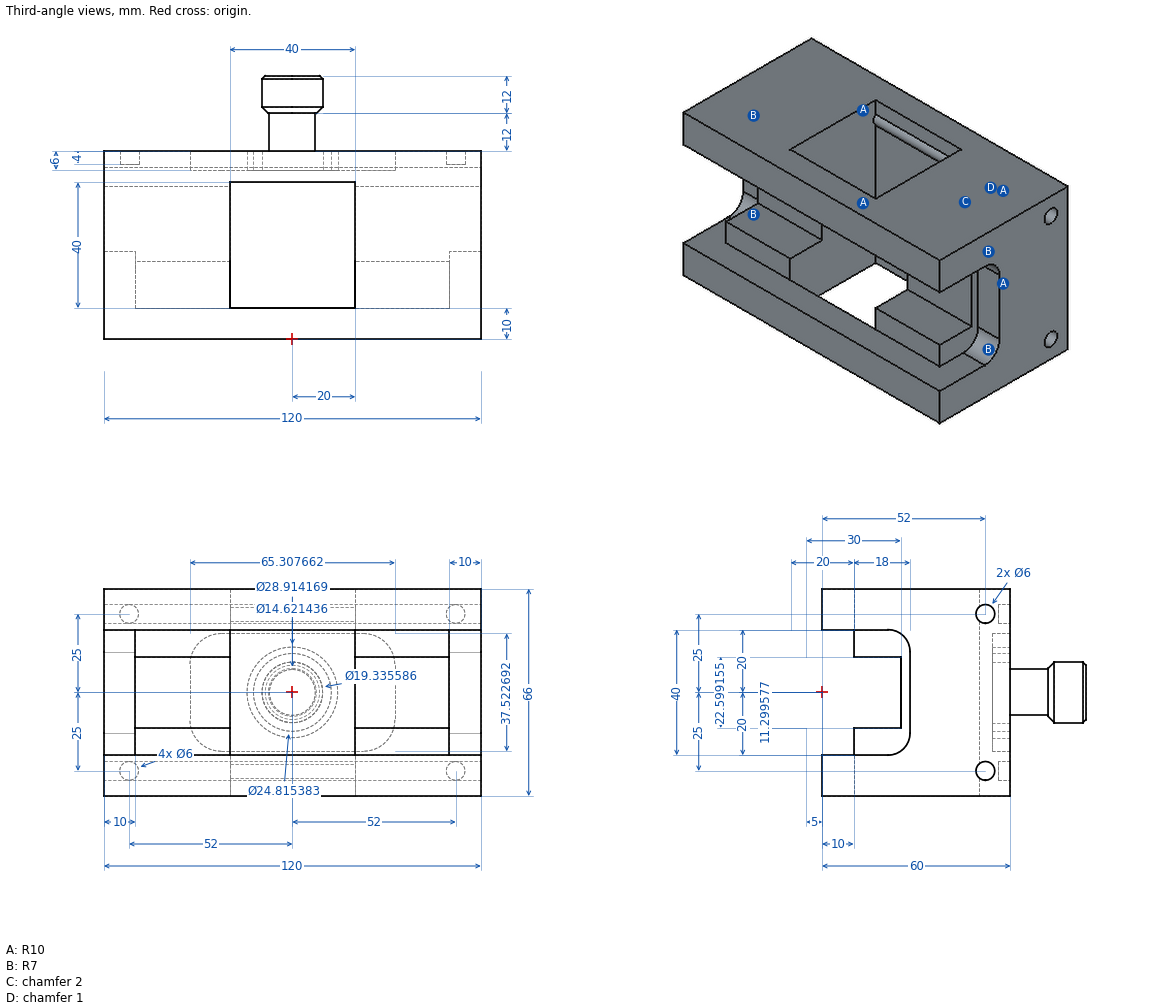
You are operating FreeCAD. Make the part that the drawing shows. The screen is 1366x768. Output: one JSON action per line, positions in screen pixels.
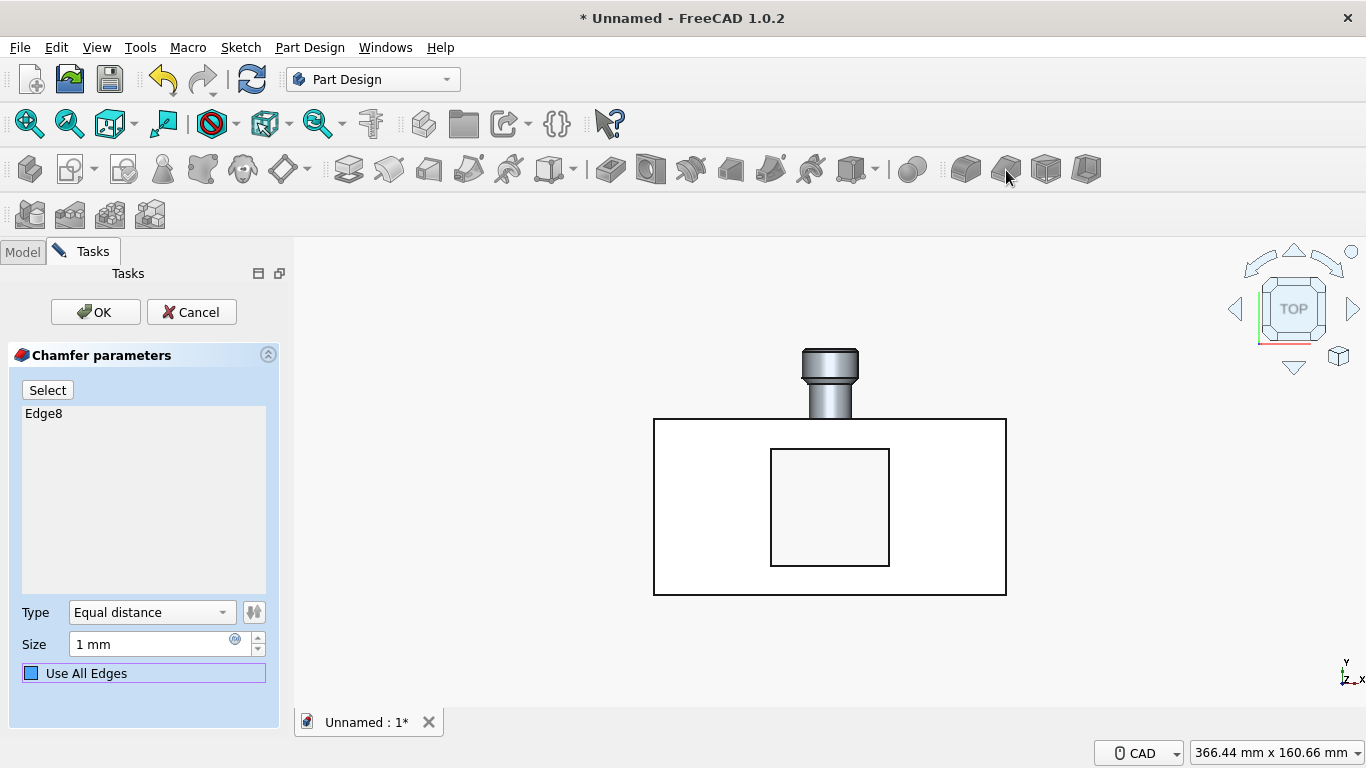
{"action": "left_click", "coordinate": [96, 312]}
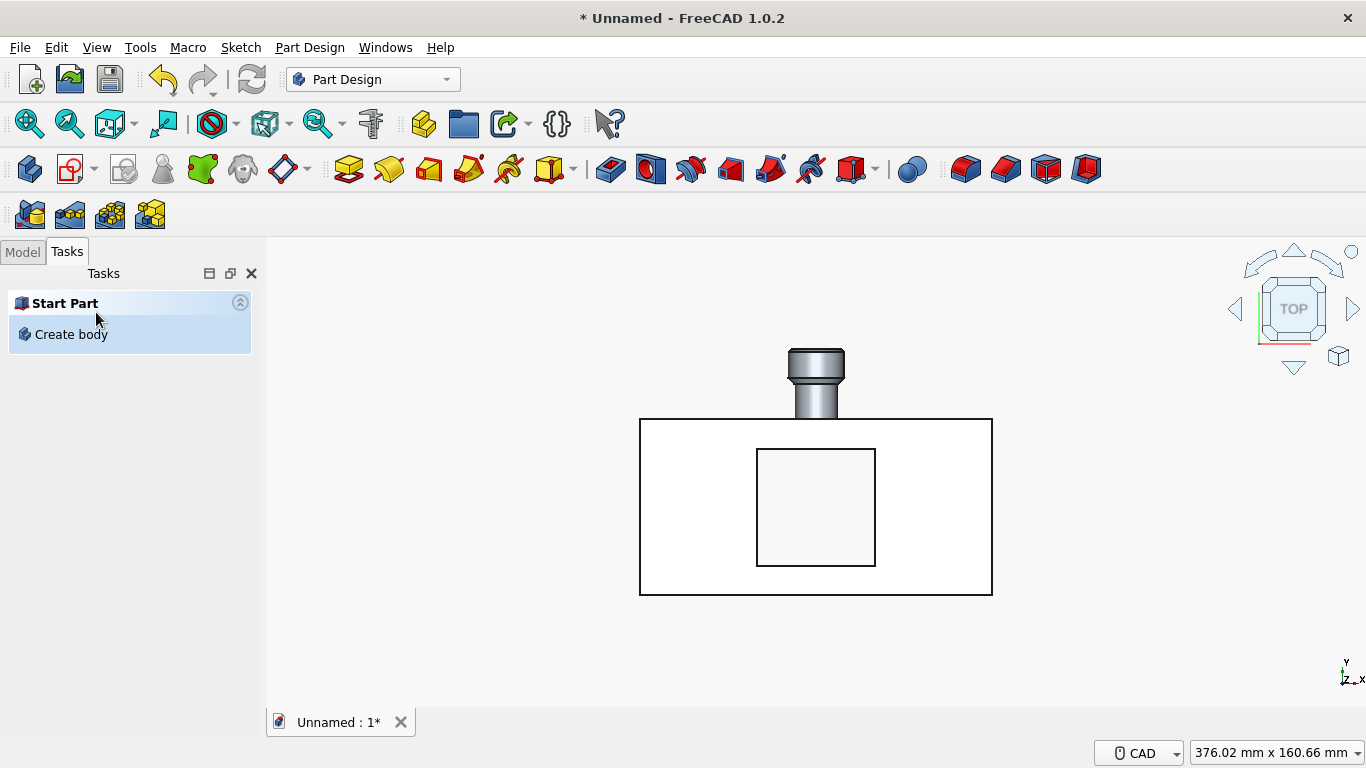
{"action": "key", "text": "0"}